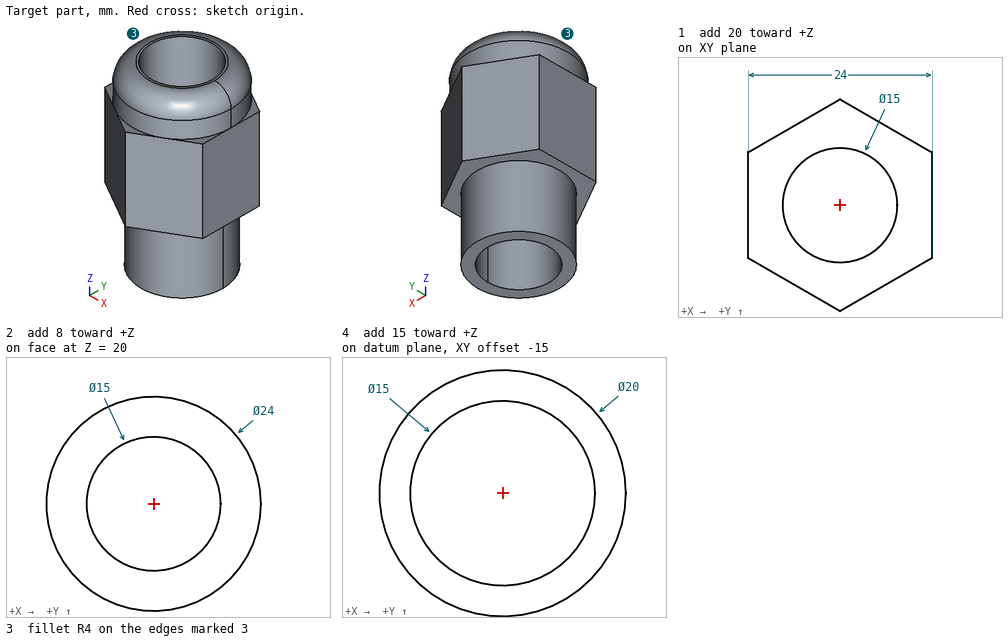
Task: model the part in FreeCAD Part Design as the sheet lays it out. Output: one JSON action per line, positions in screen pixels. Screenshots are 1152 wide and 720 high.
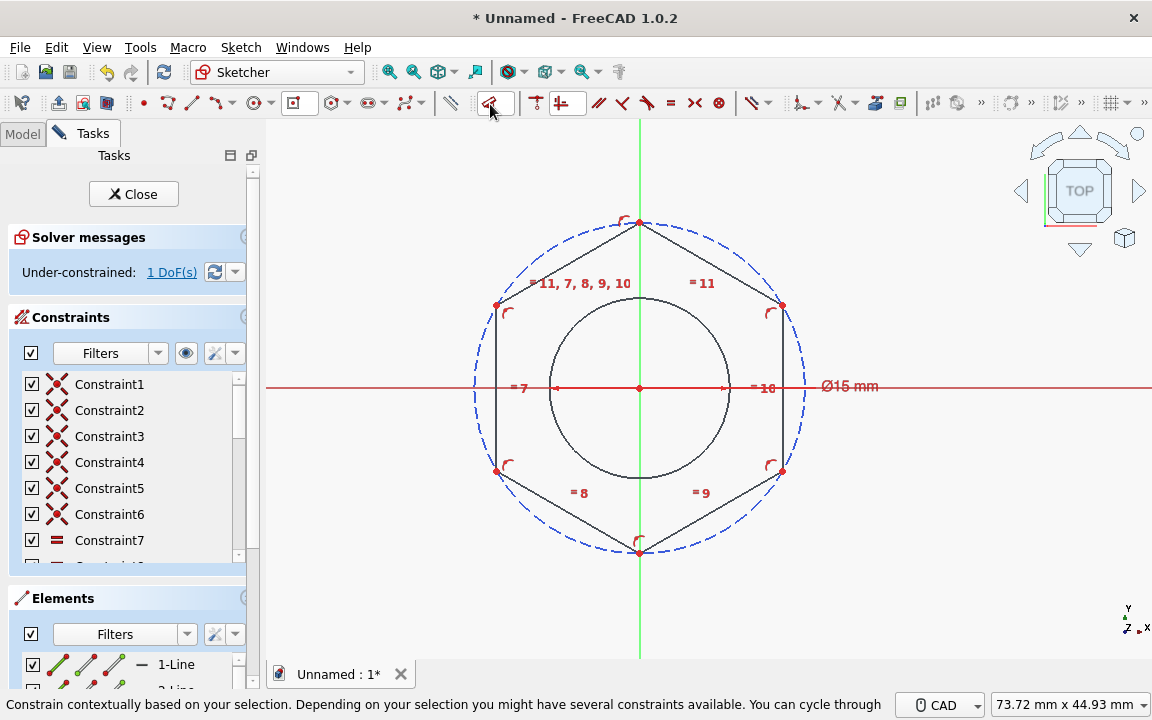
{"action": "left_click", "coordinate": [496, 306]}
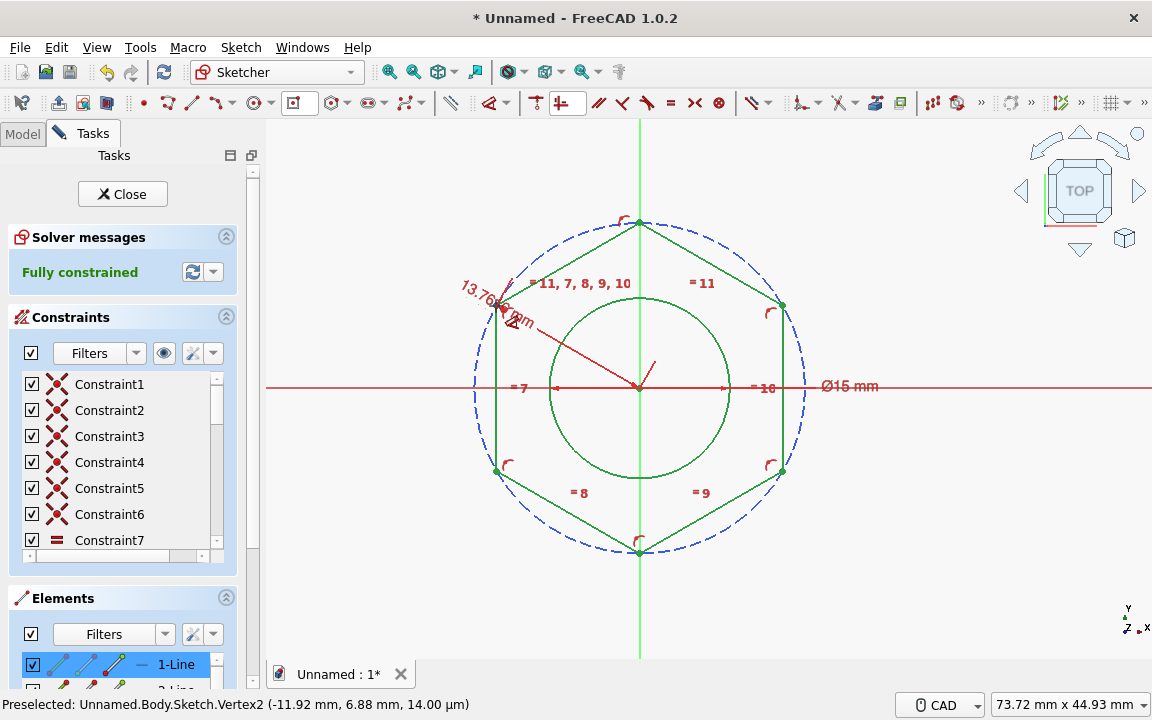
{"action": "left_click", "coordinate": [783, 471]}
{"action": "left_click", "coordinate": [539, 553]}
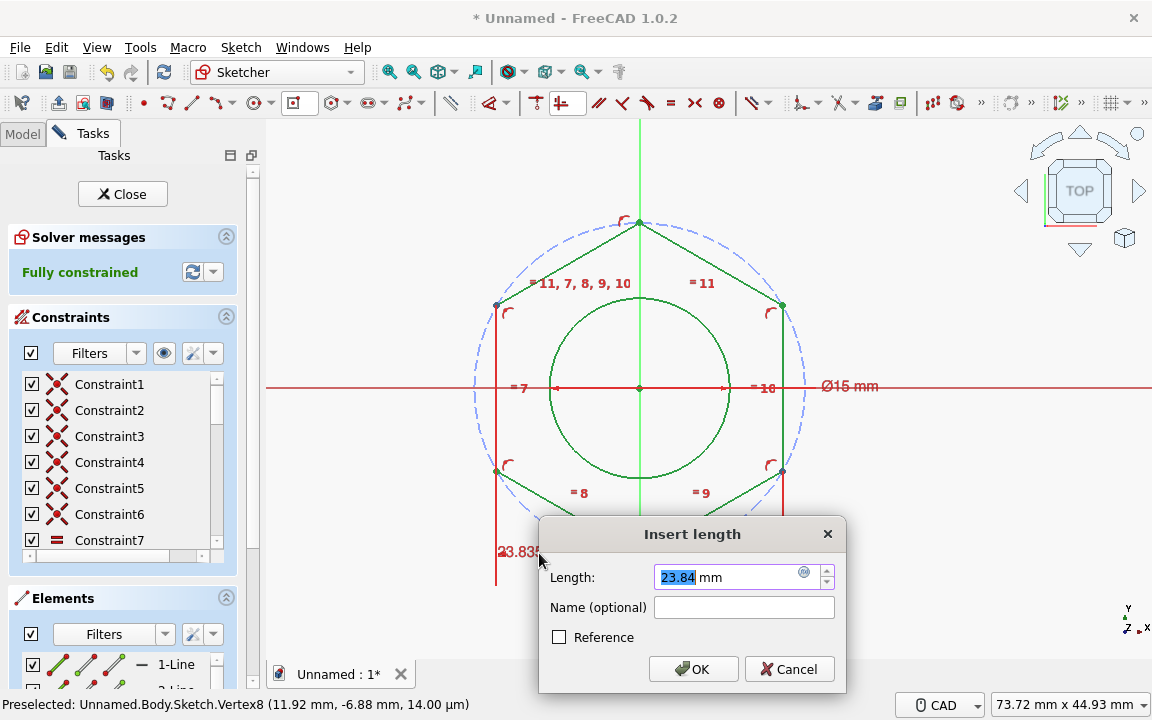
{"action": "type", "text": "24"}
{"action": "key", "text": "Return"}
{"action": "key", "text": "Escape"}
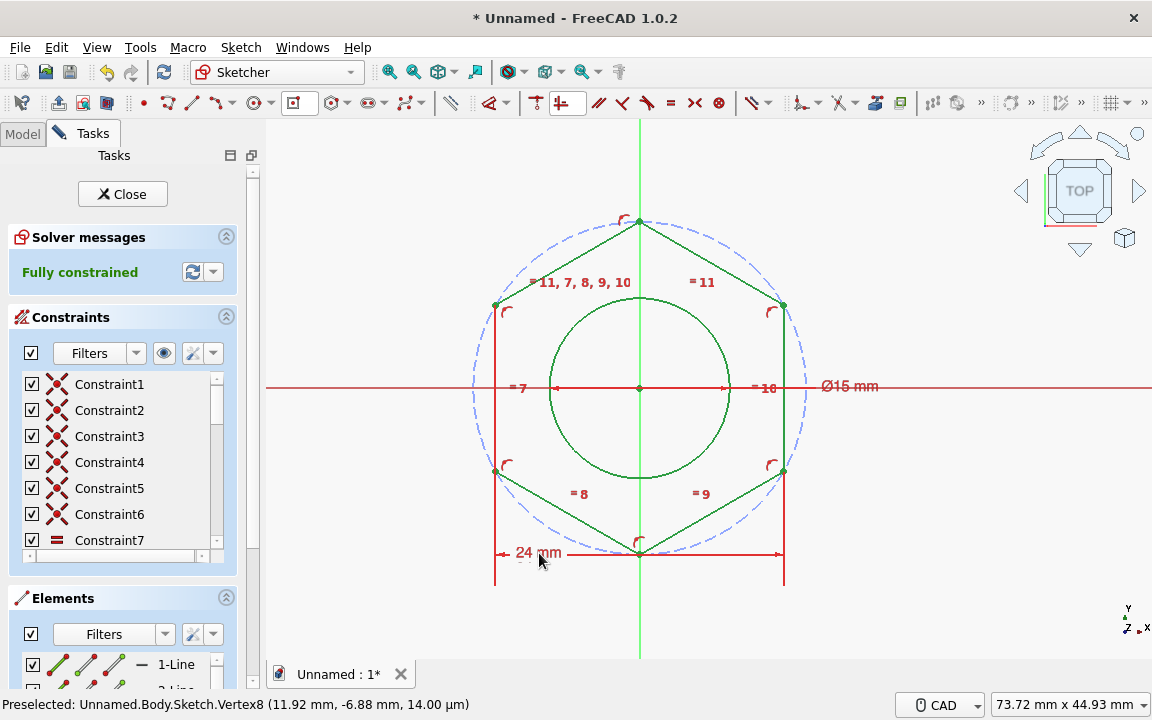
{"action": "left_click", "coordinate": [123, 194]}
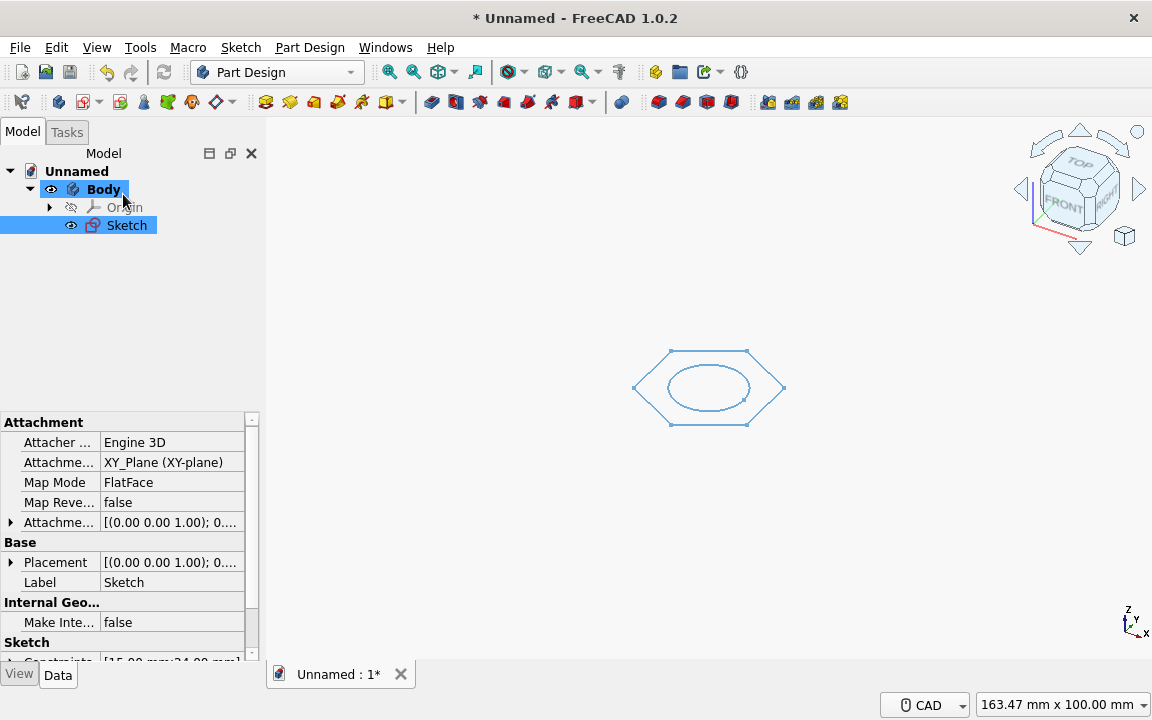
{"action": "left_click", "coordinate": [266, 102]}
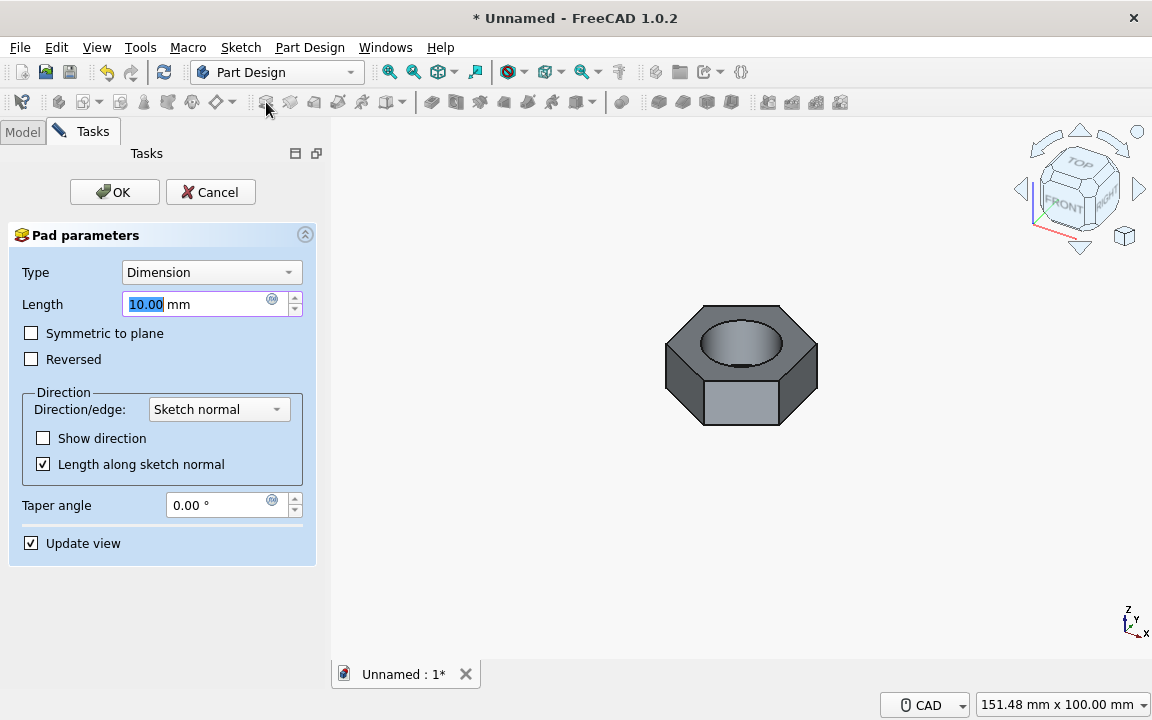
{"action": "type", "text": "20"}
{"action": "key", "text": "Tab"}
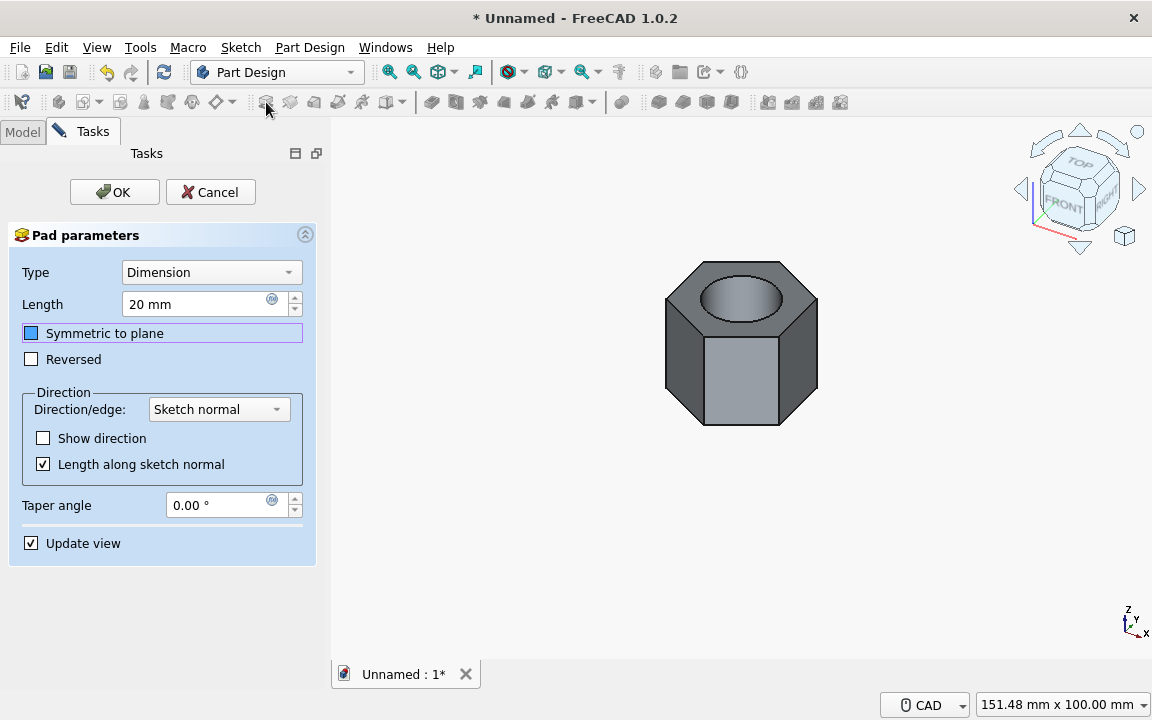
{"action": "left_click", "coordinate": [115, 192]}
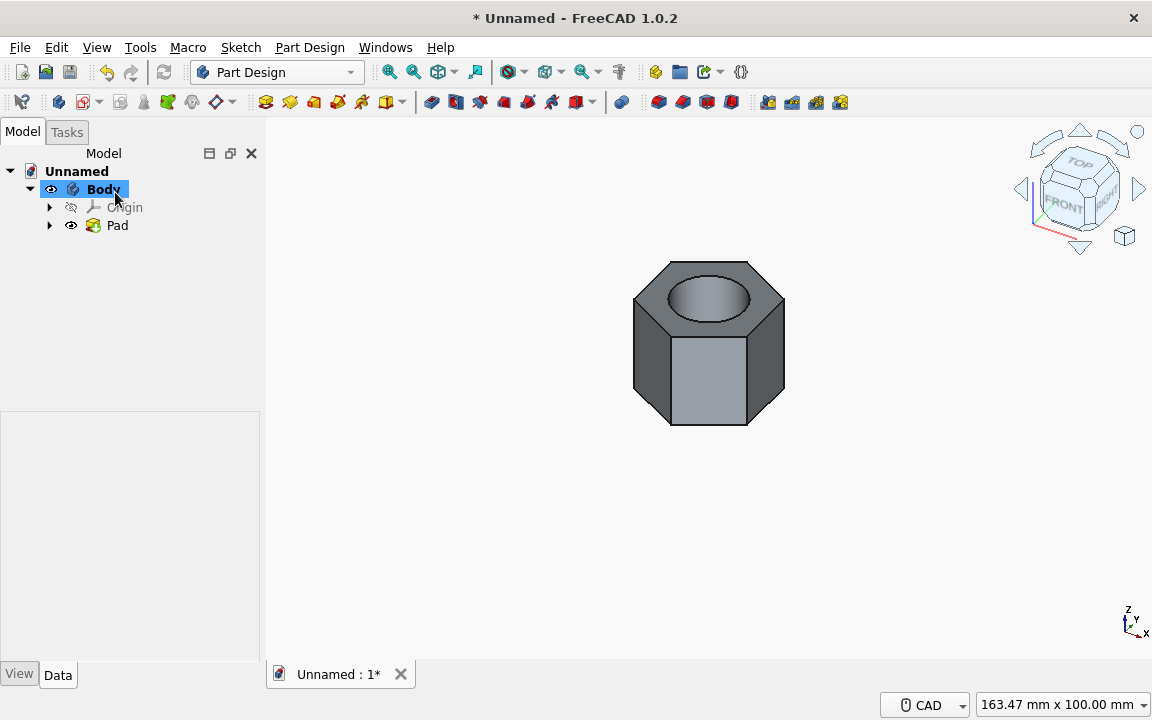
{"action": "key", "text": "v f"}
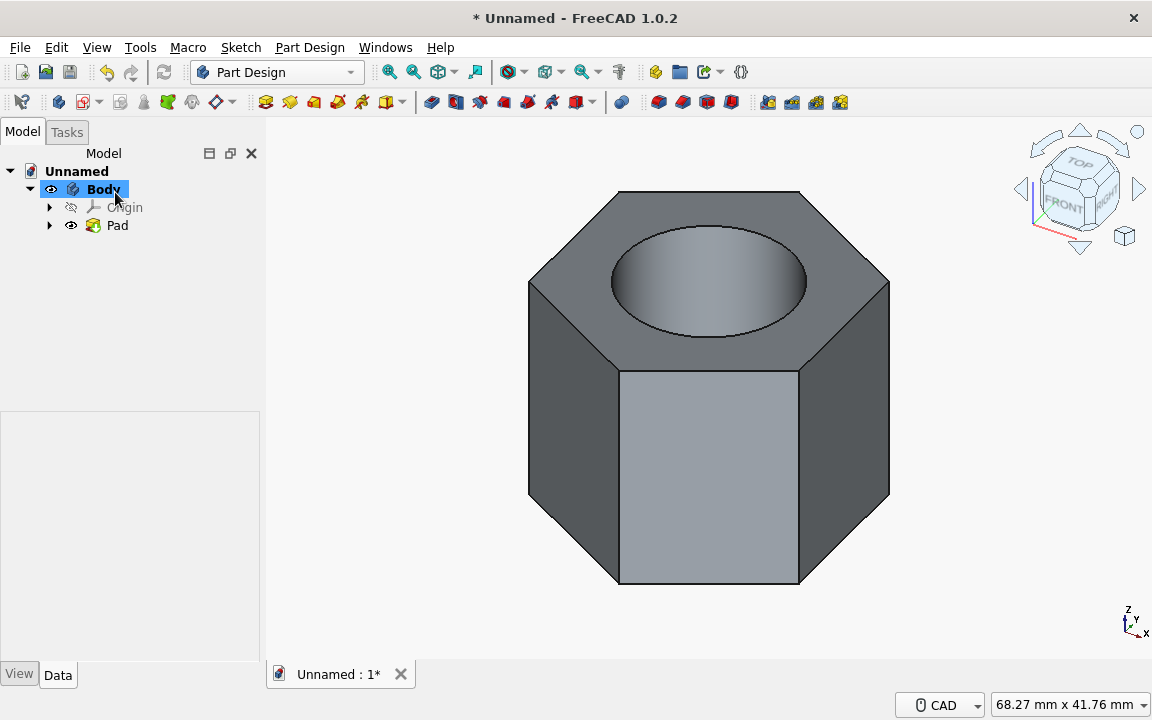
{"action": "left_click", "coordinate": [837, 255]}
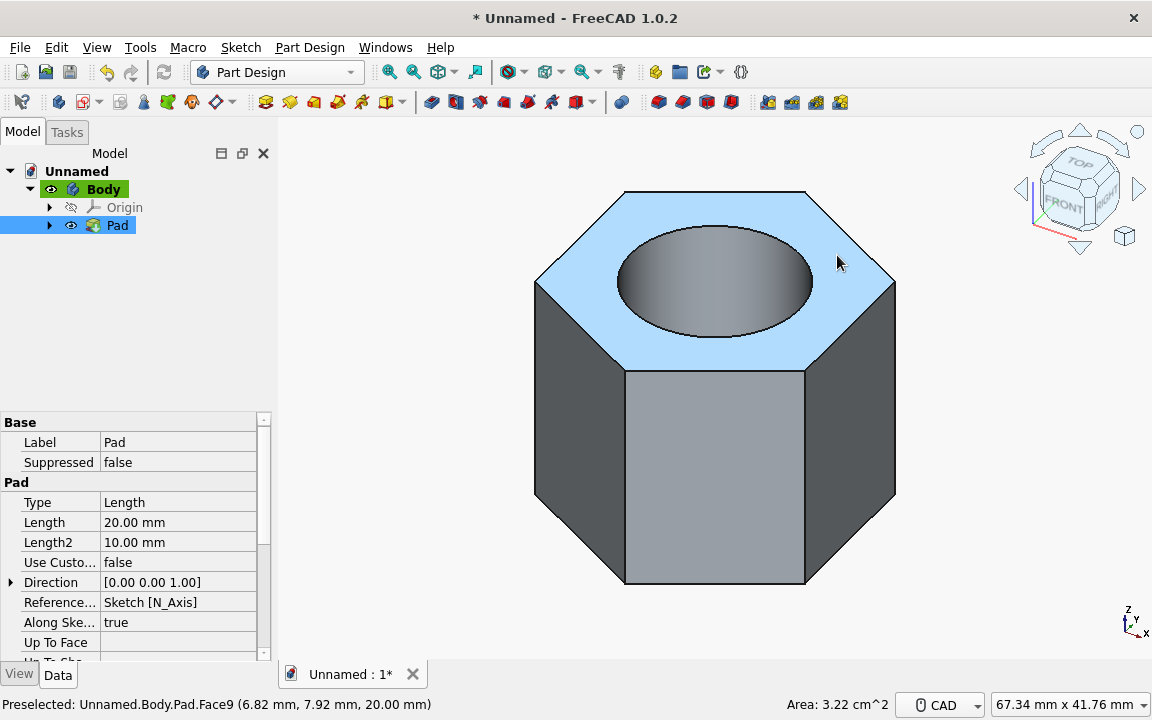
{"action": "left_click", "coordinate": [84, 102]}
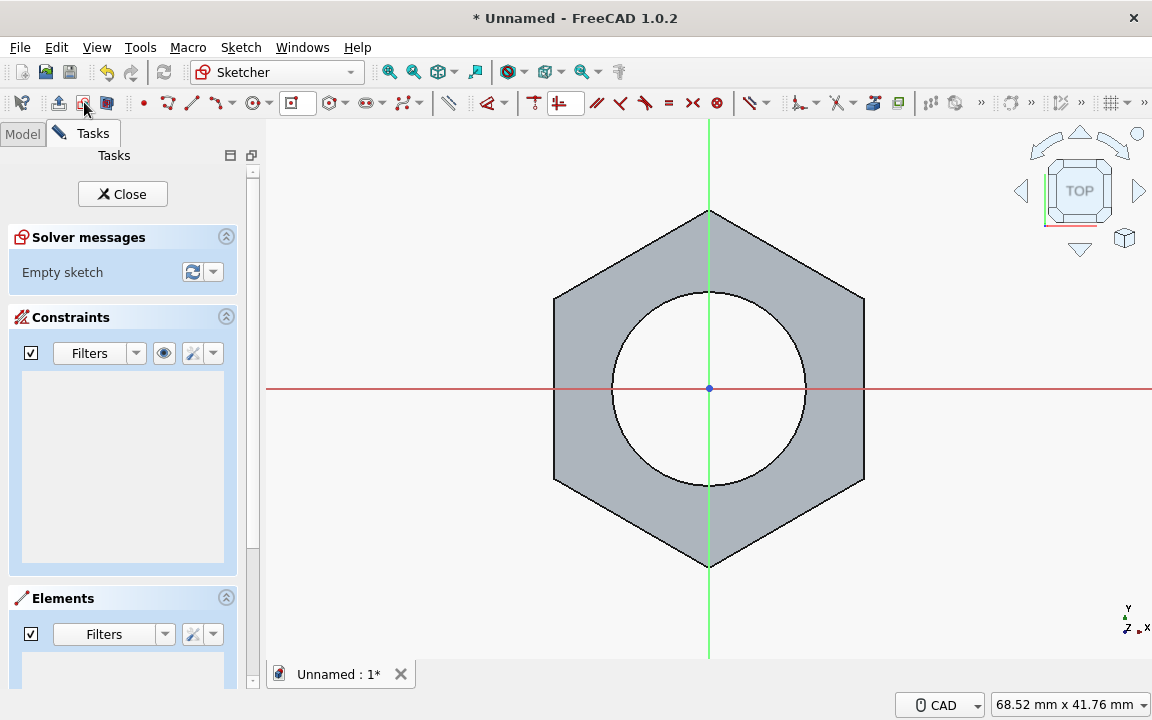
{"action": "left_click", "coordinate": [254, 104]}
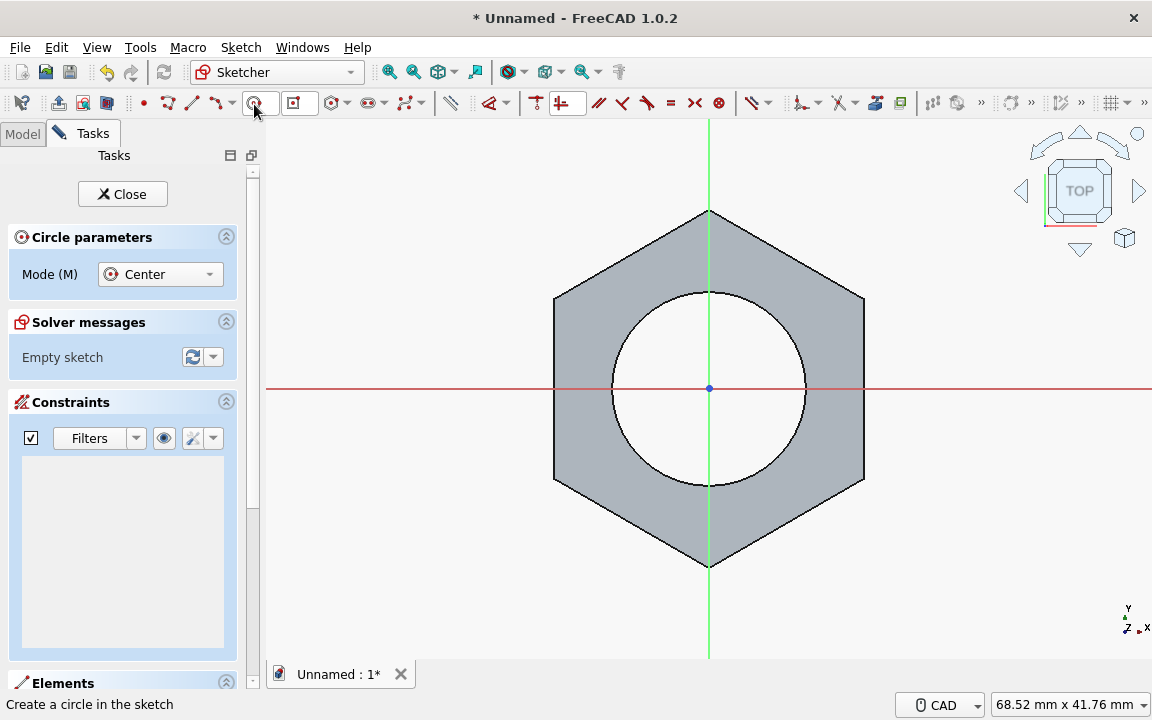
{"action": "left_click", "coordinate": [709, 389]}
{"action": "mouse_move", "coordinate": [819, 279]}